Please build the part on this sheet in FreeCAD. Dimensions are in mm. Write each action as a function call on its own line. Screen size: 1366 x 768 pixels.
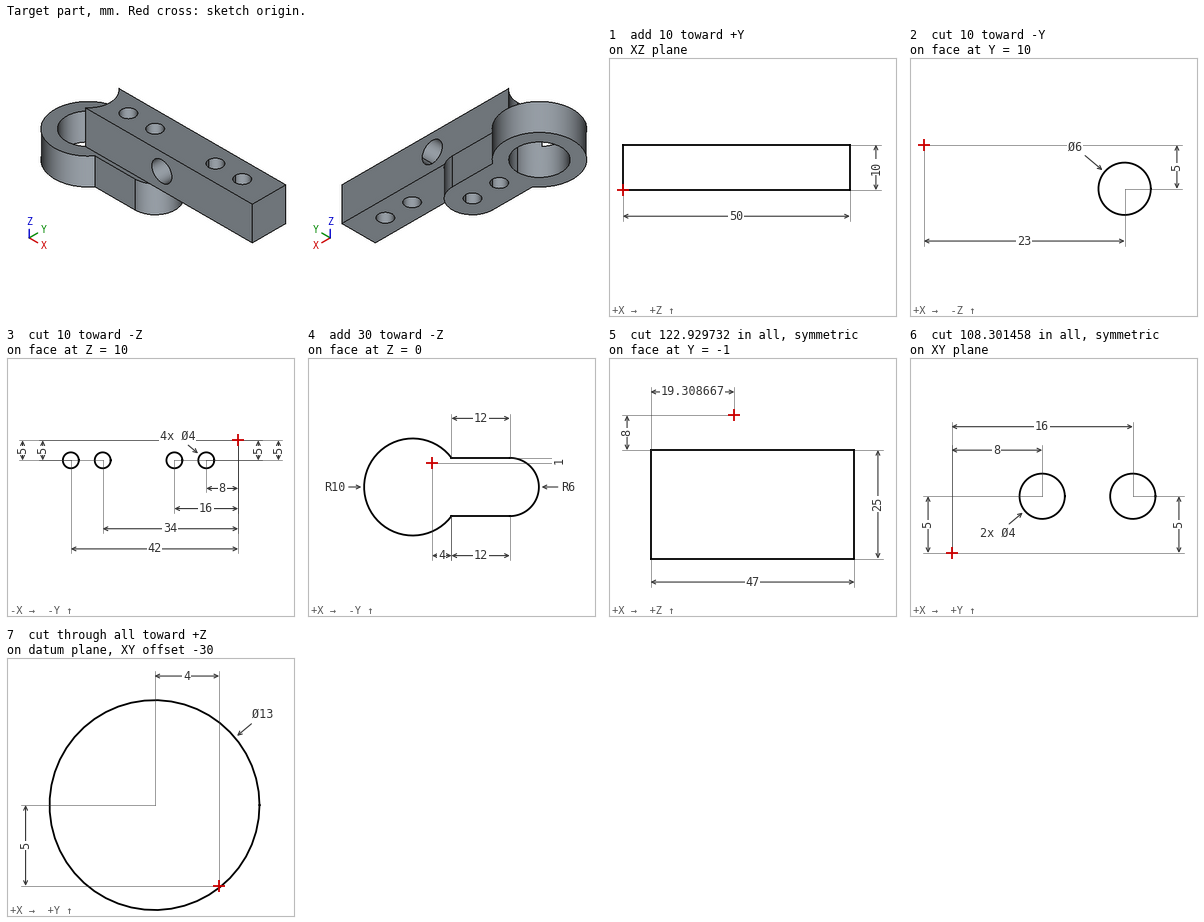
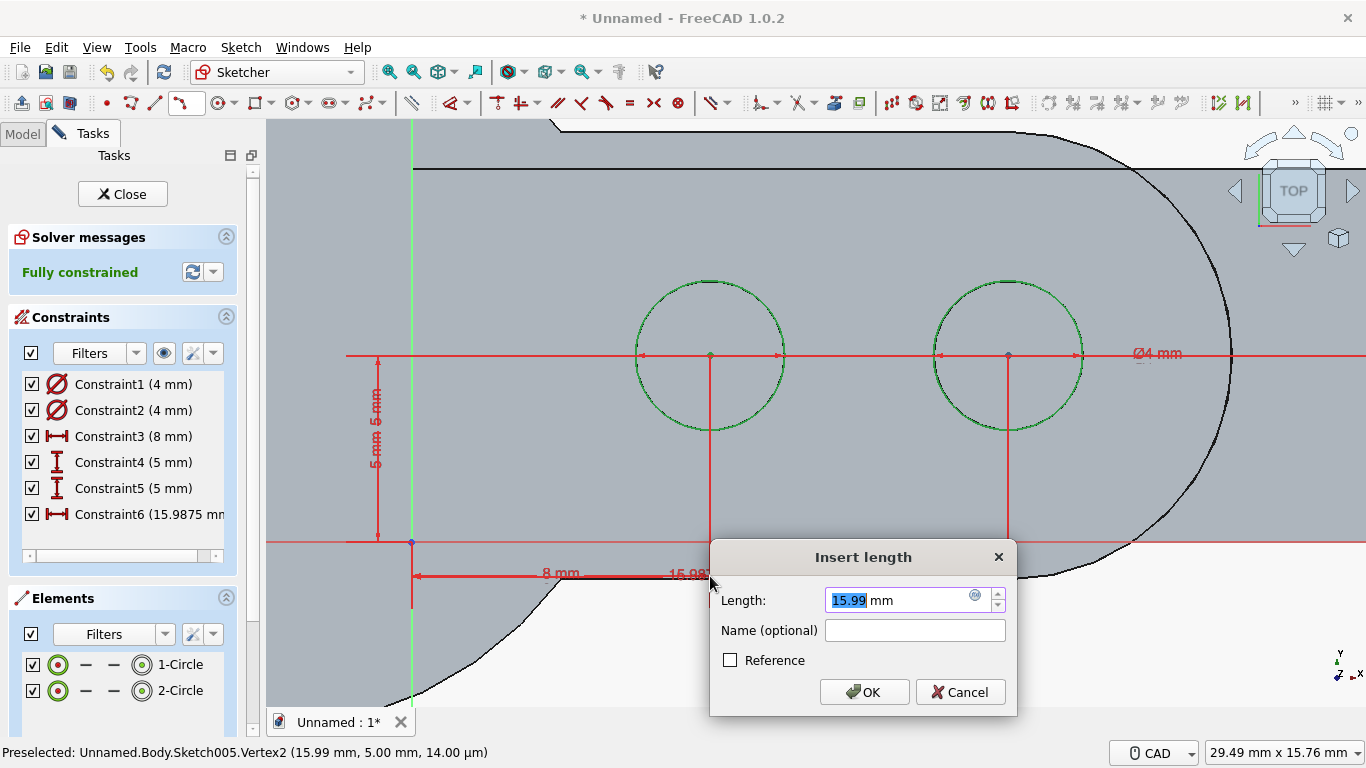
text(16)
key(Return)
key(Escape)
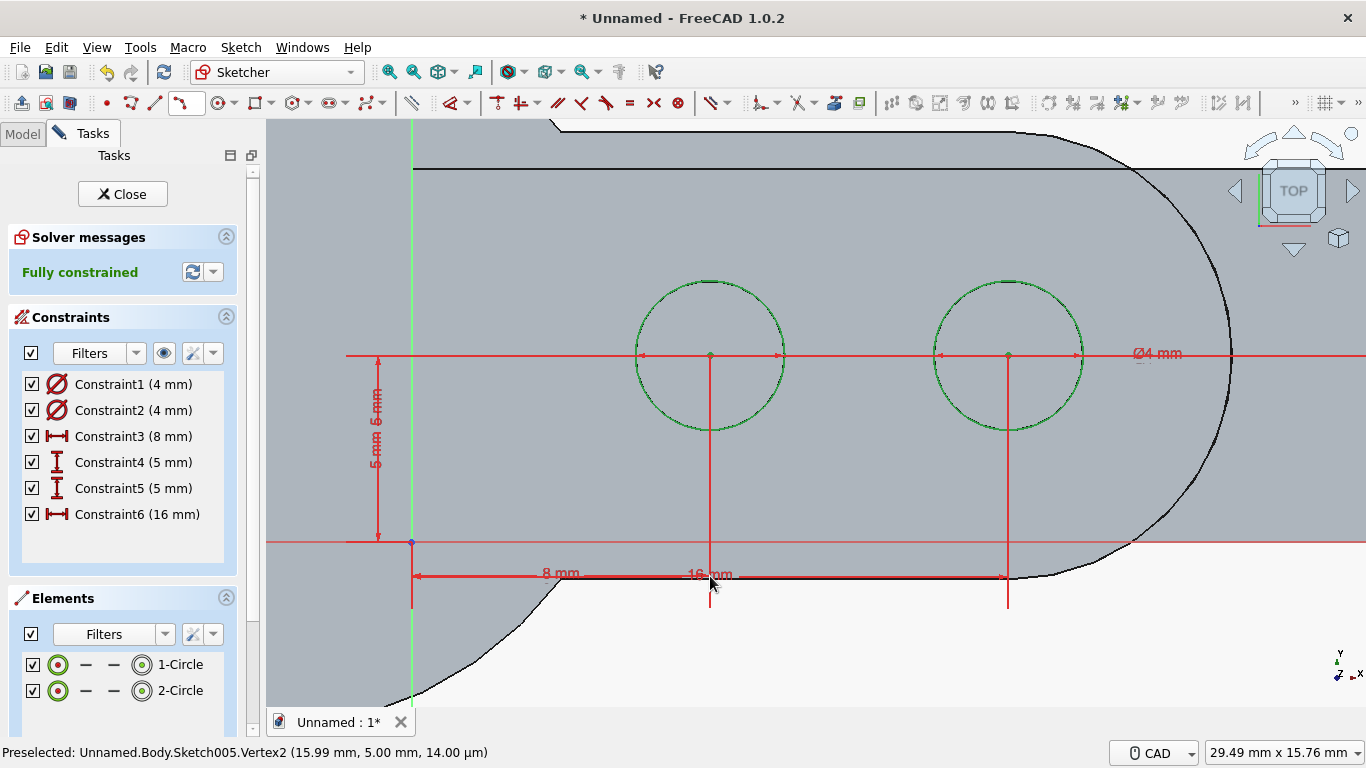
click(123, 194)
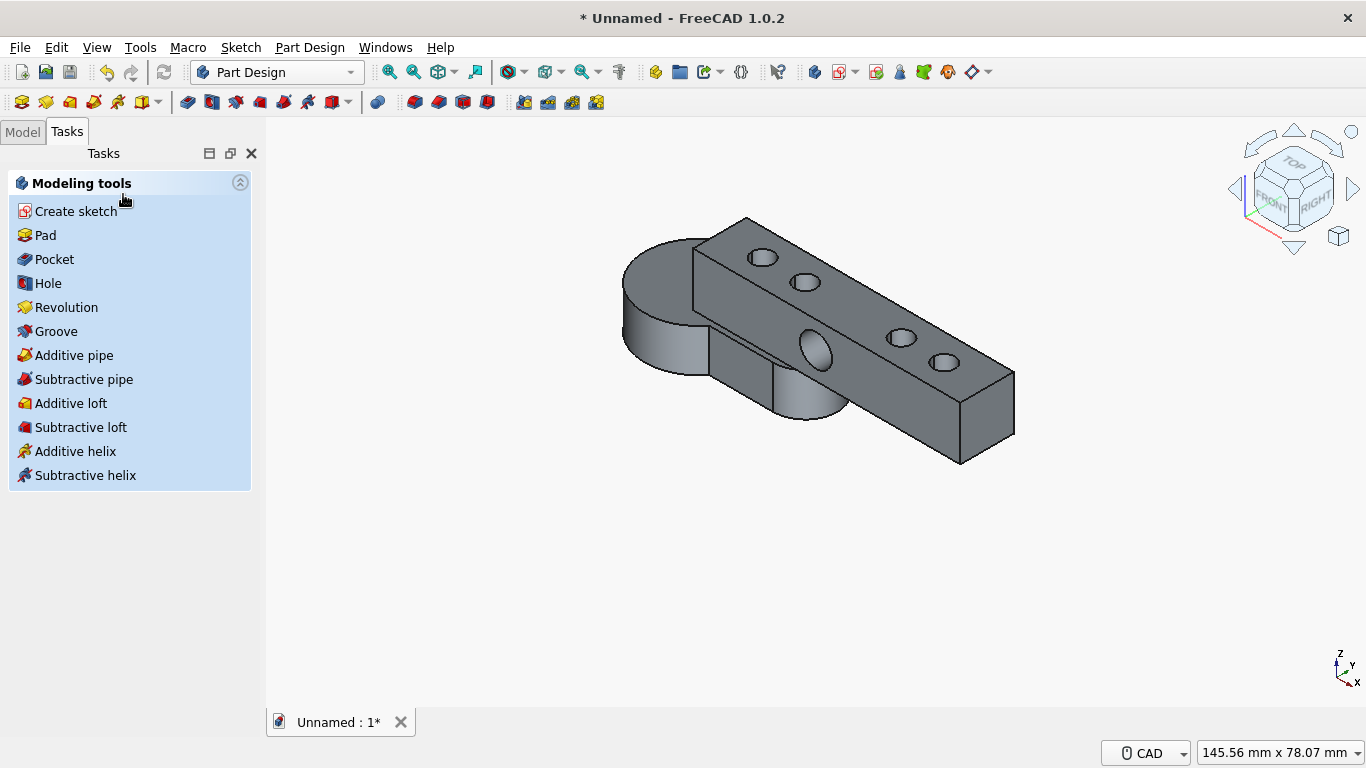
click(188, 102)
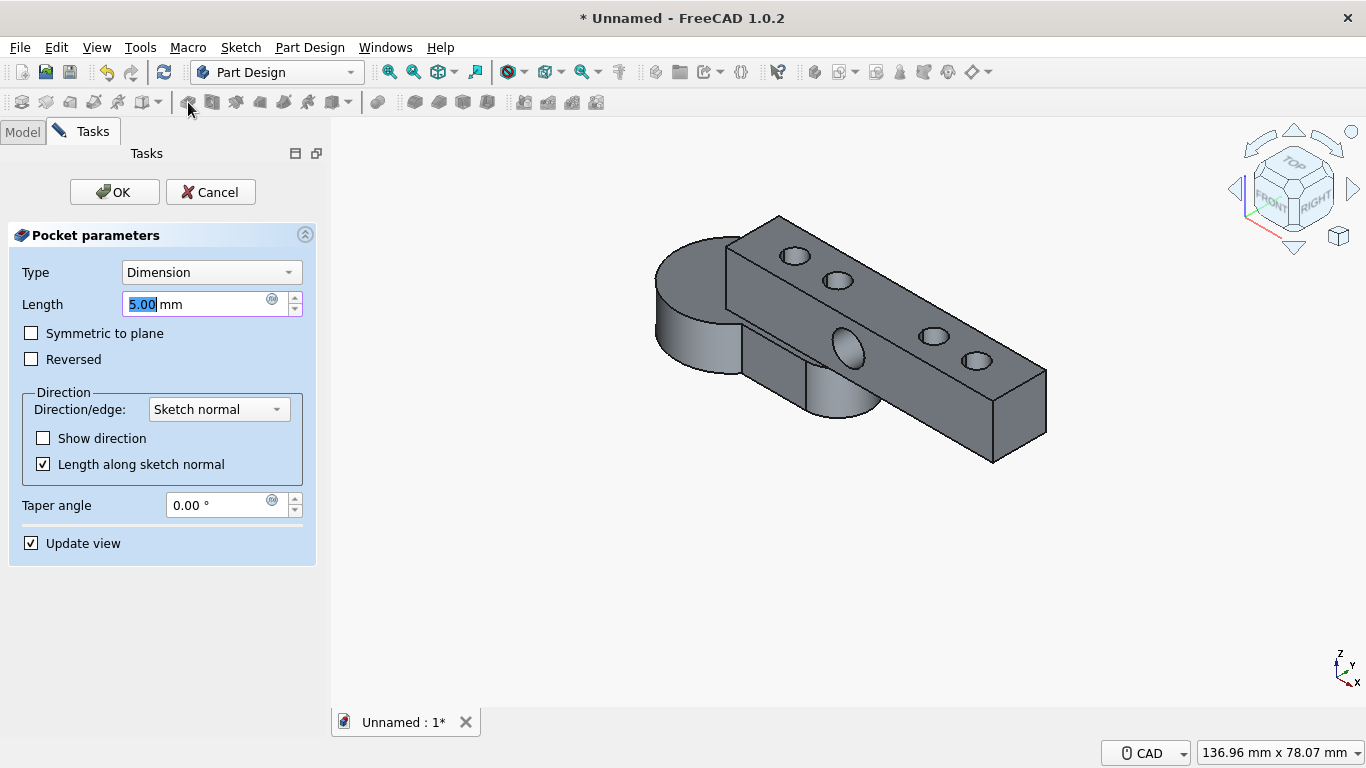
text(108.301458)
key(Tab)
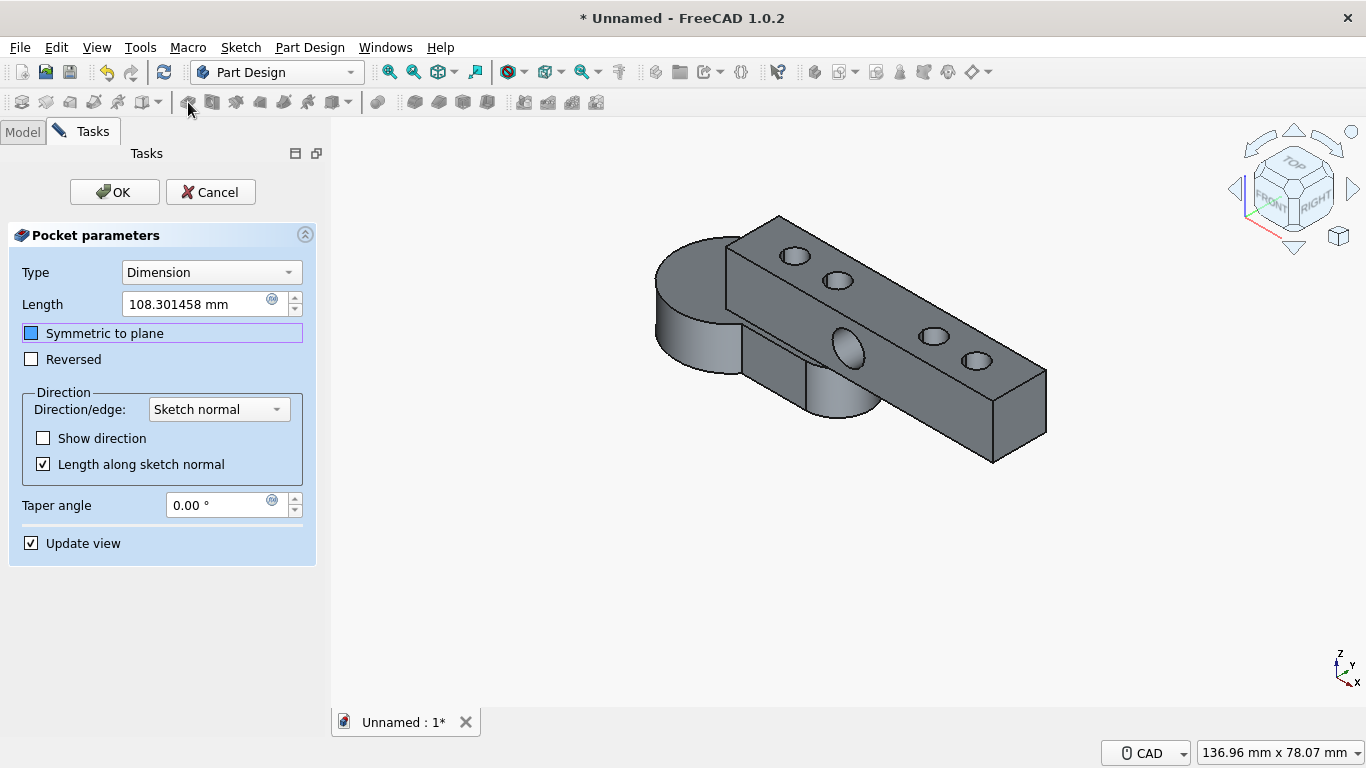
click(30, 333)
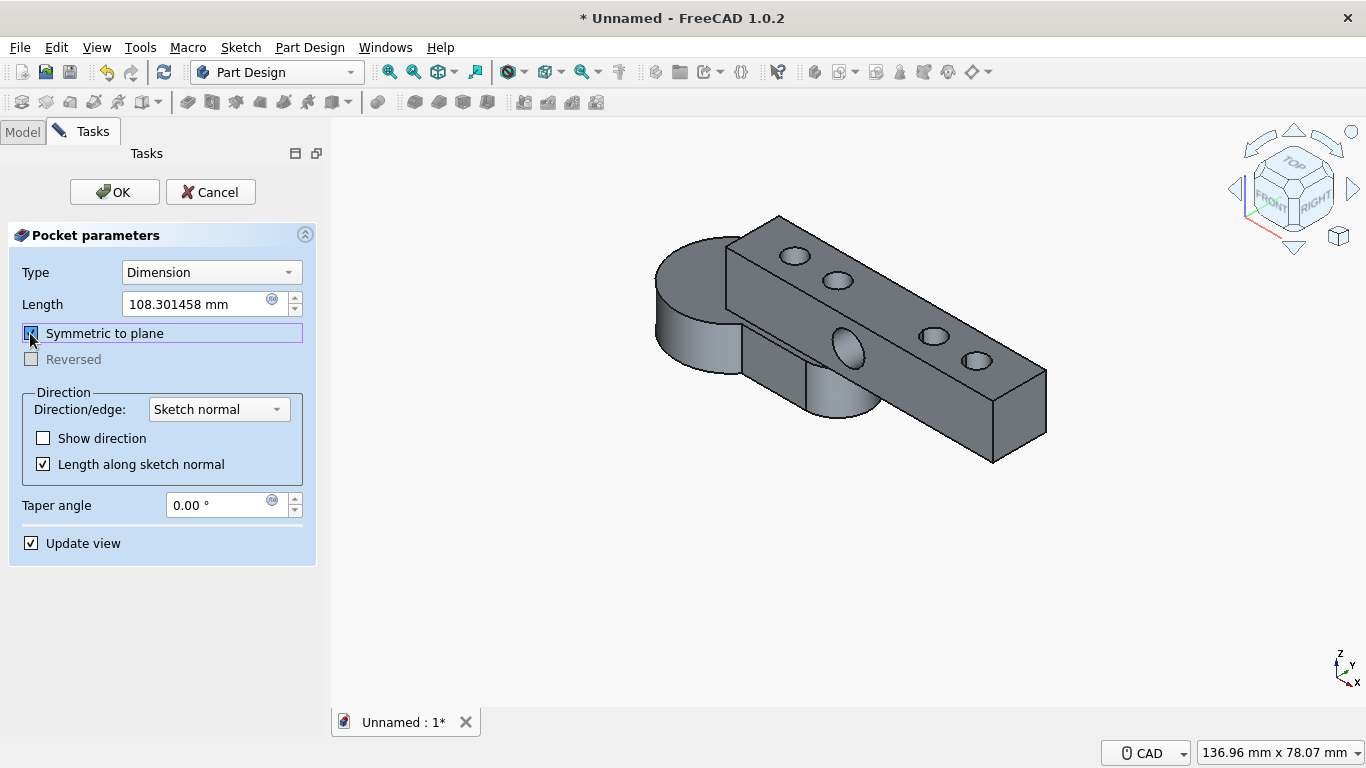
click(115, 192)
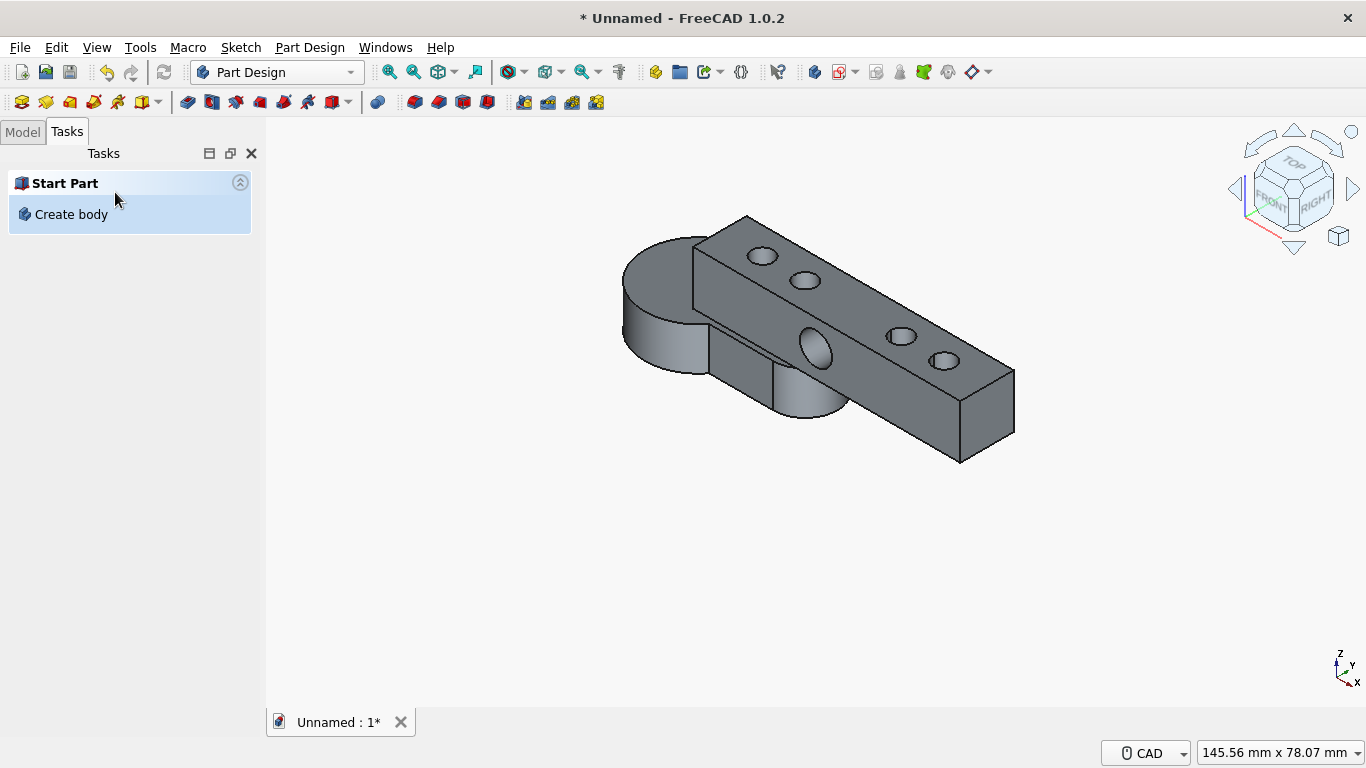
click(23, 131)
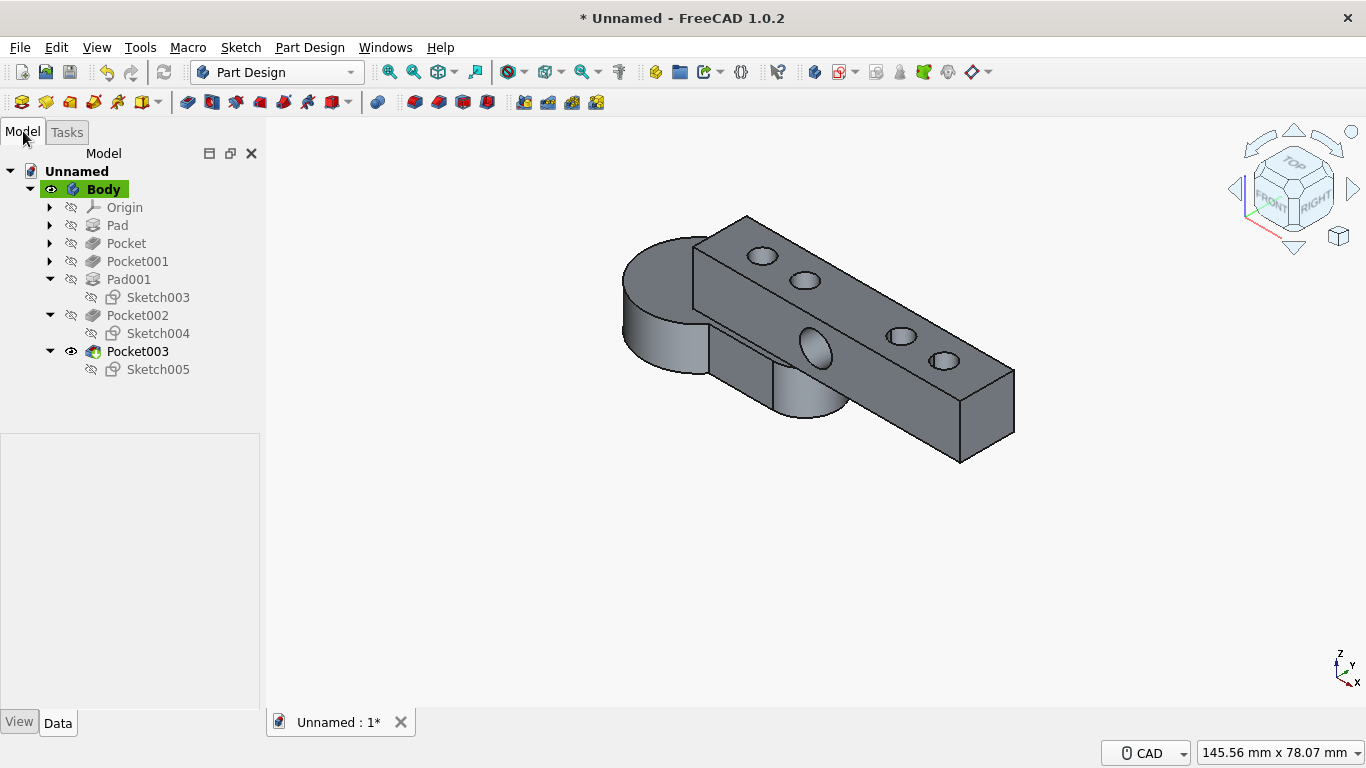
click(50, 207)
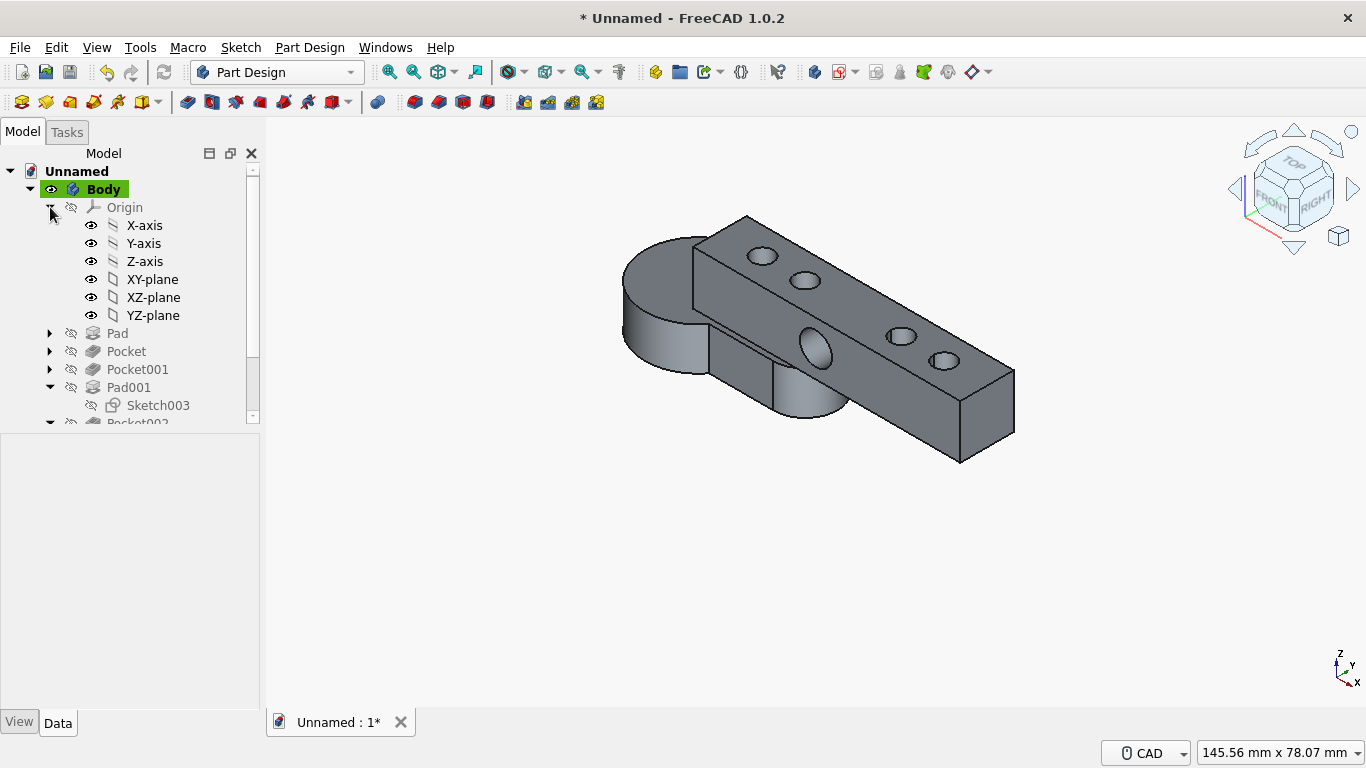
click(136, 279)